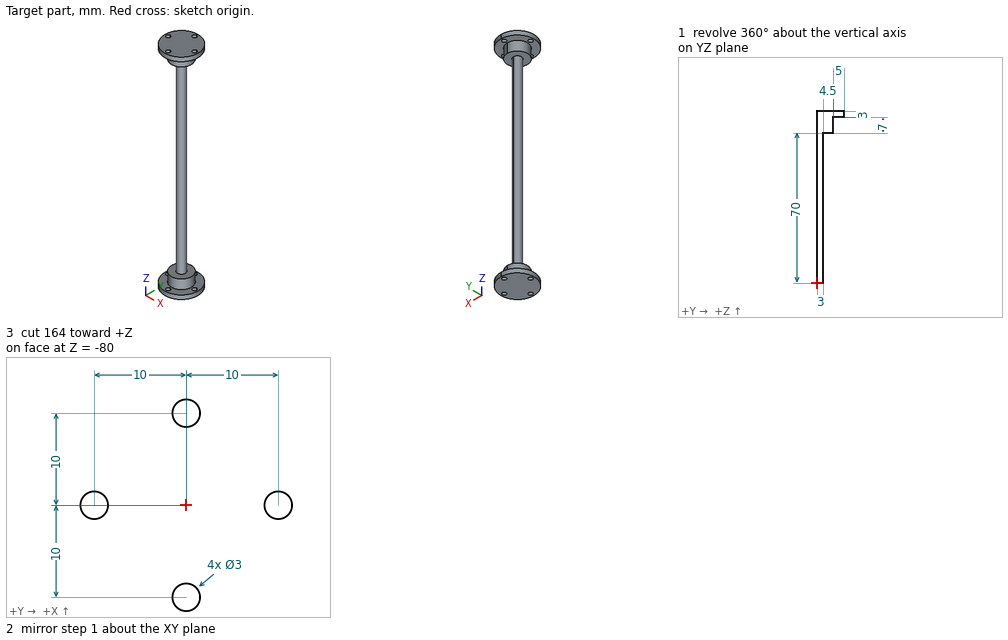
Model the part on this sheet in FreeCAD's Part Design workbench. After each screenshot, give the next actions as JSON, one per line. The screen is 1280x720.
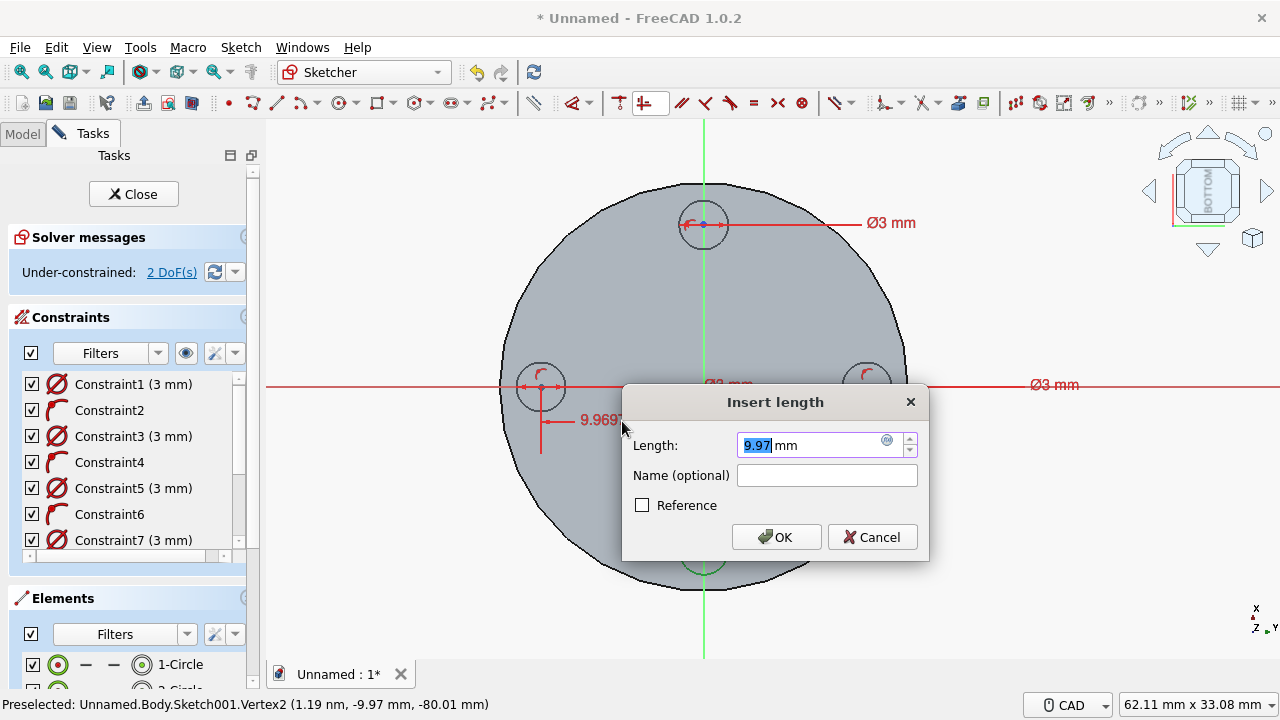
{"action": "type", "text": "10"}
{"action": "key", "text": "Return"}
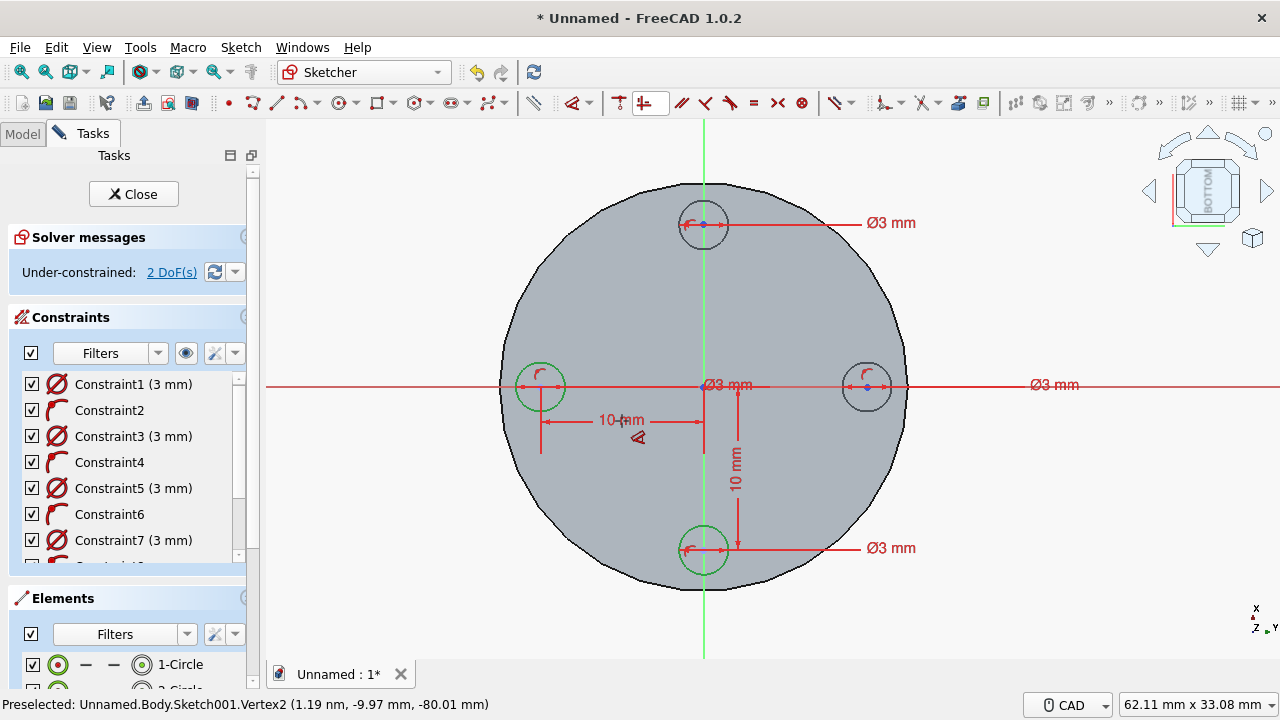
{"action": "left_click", "coordinate": [704, 225]}
{"action": "left_click", "coordinate": [738, 306]}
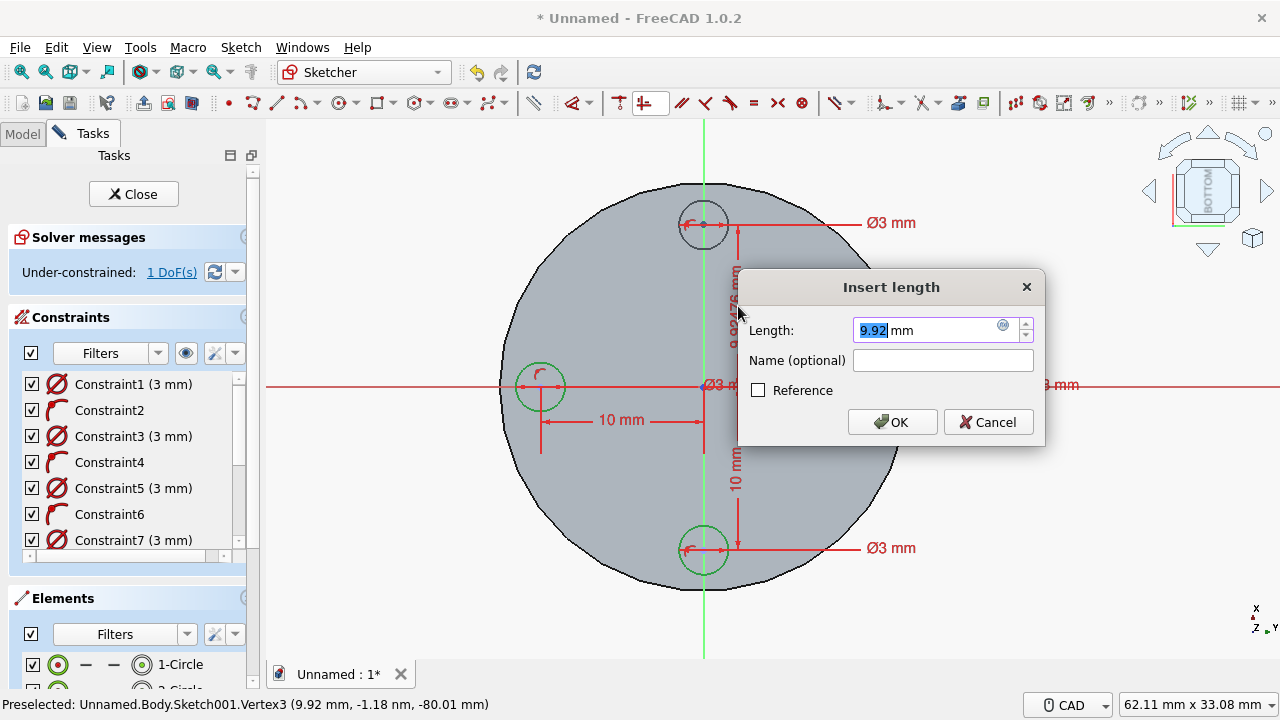
{"action": "type", "text": "10"}
{"action": "key", "text": "Return"}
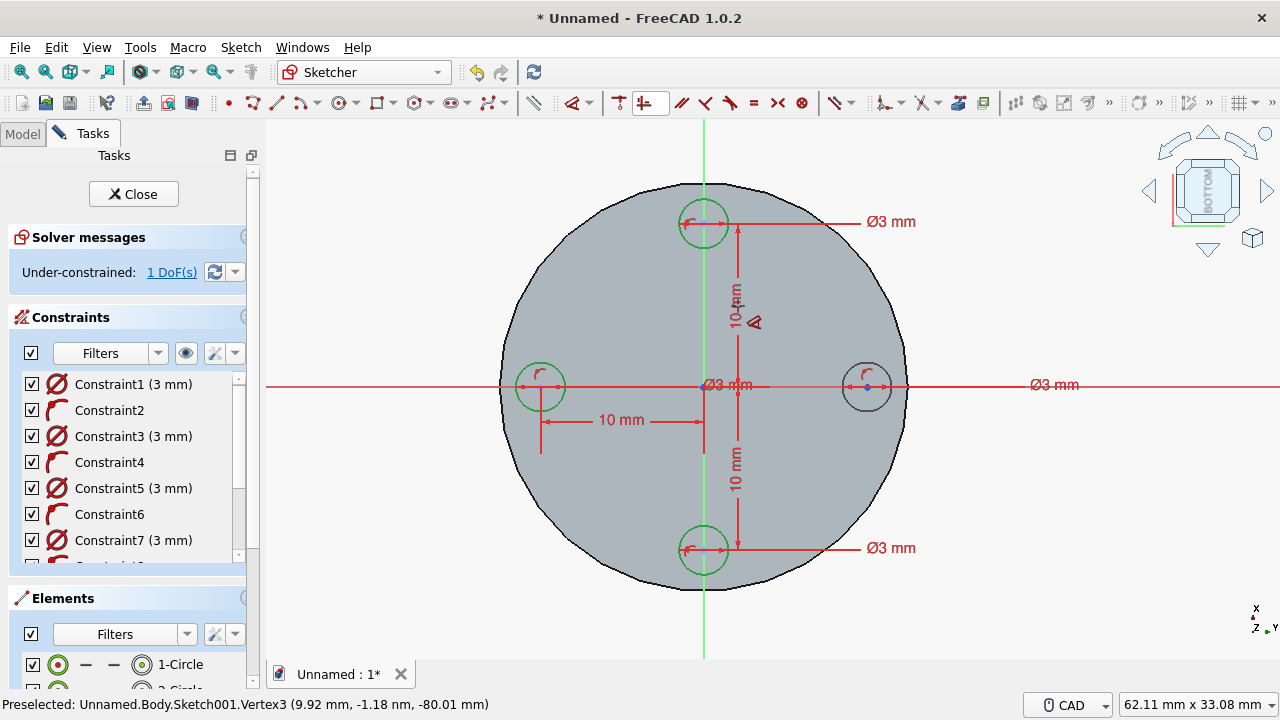
{"action": "left_click", "coordinate": [867, 387]}
{"action": "left_click", "coordinate": [785, 353]}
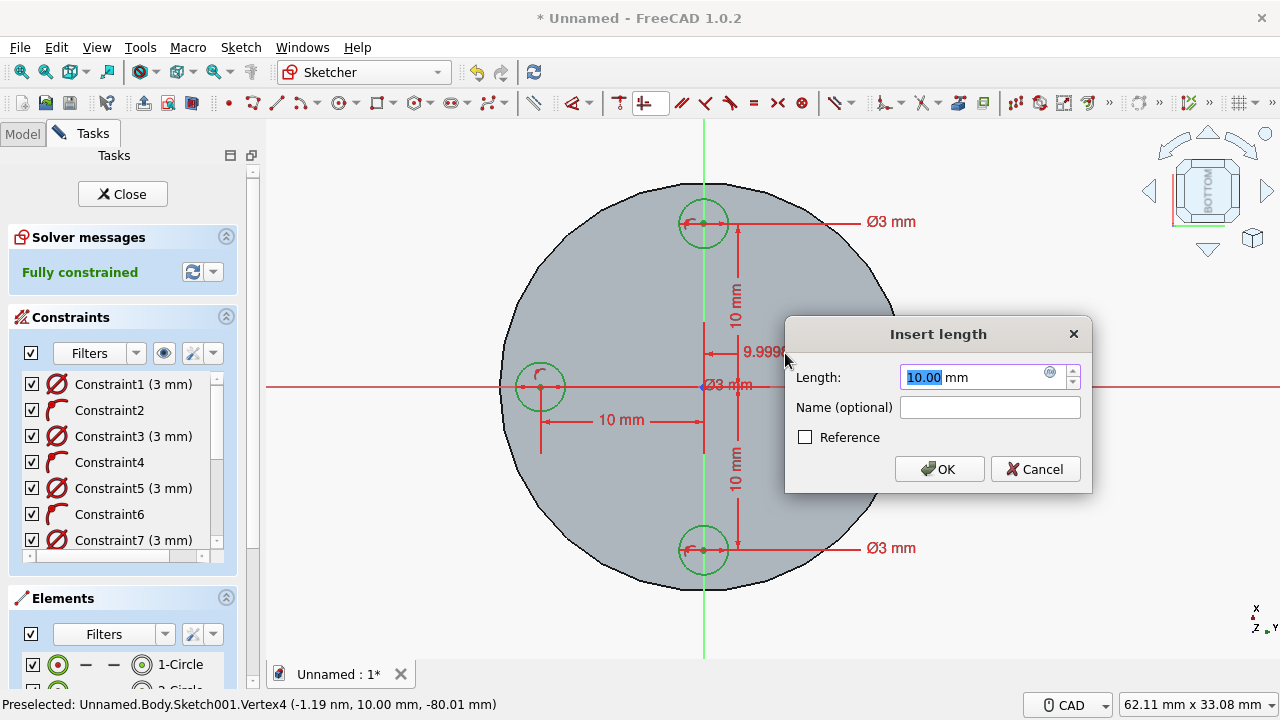
{"action": "type", "text": "10"}
{"action": "key", "text": "Return"}
{"action": "key", "text": "Escape"}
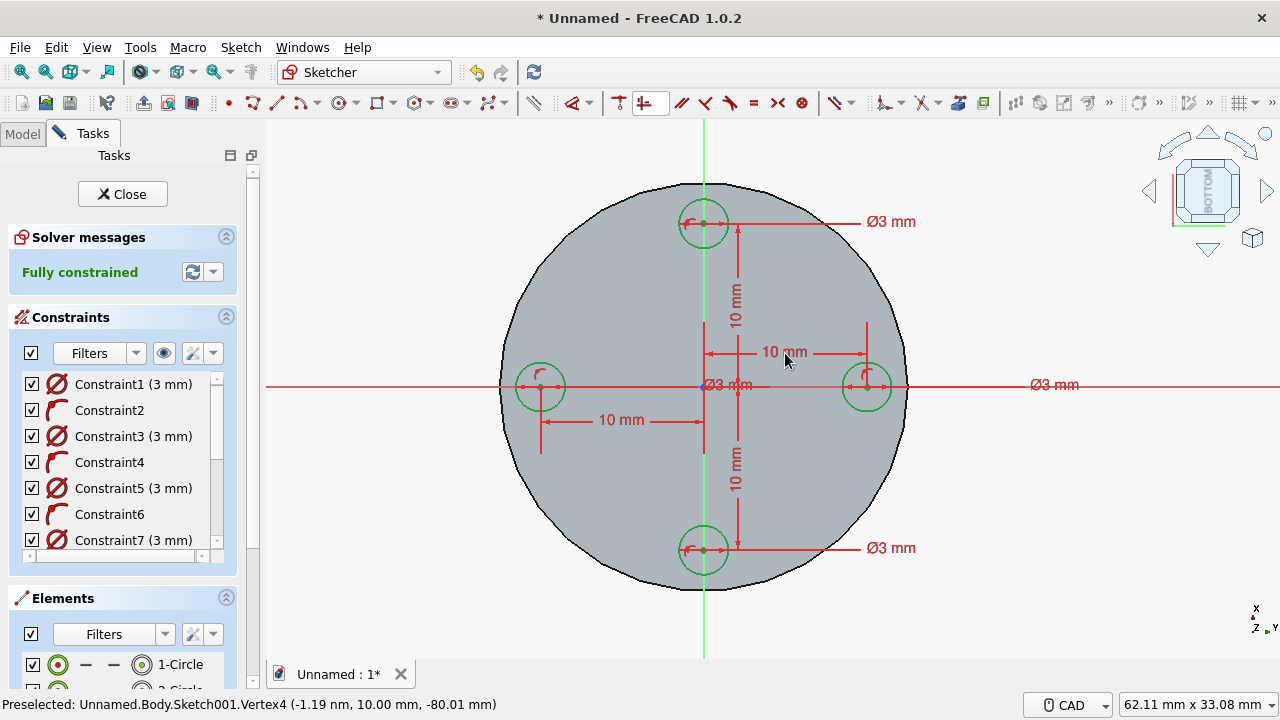
{"action": "left_click", "coordinate": [123, 194]}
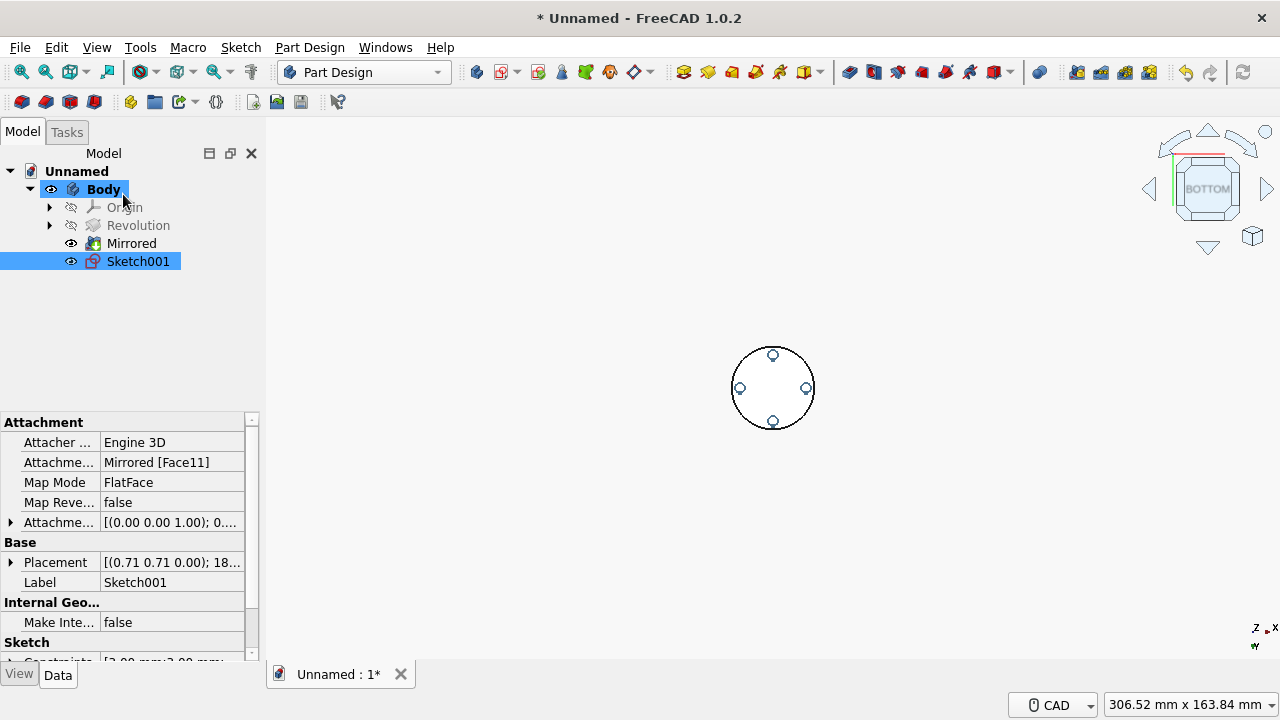
{"action": "left_click", "coordinate": [850, 72]}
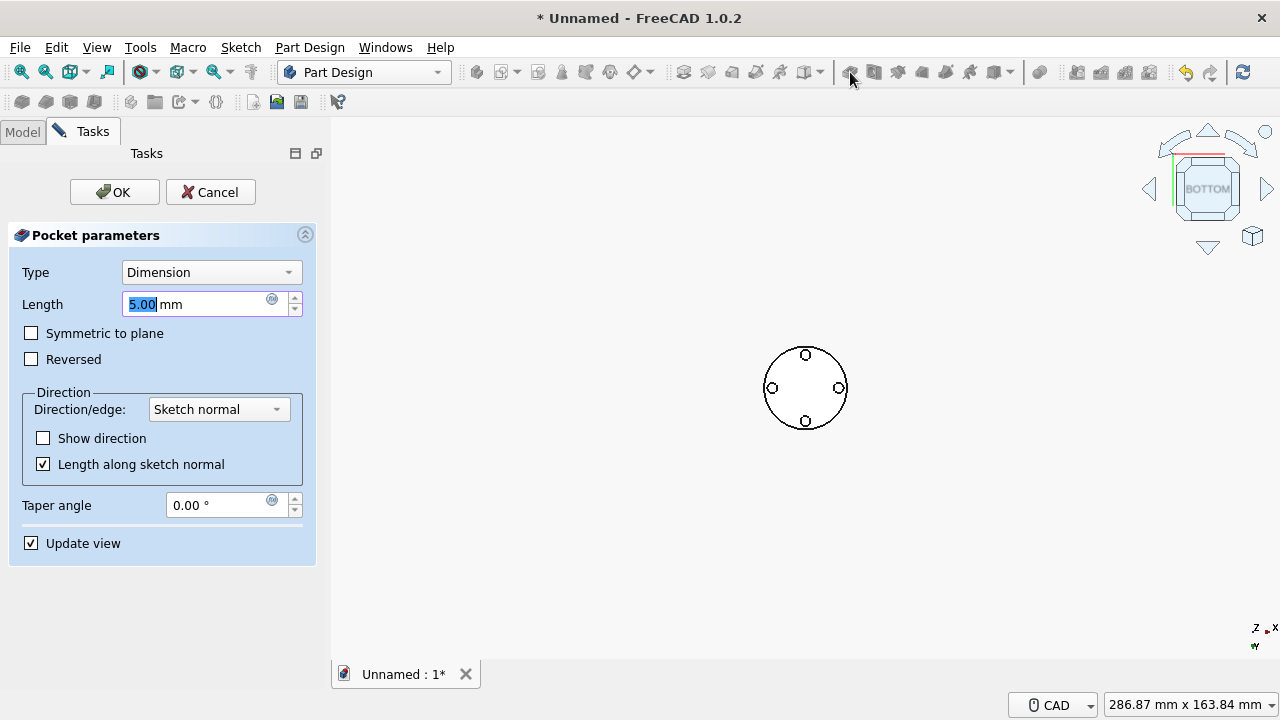
{"action": "type", "text": "164"}
{"action": "key", "text": "Tab"}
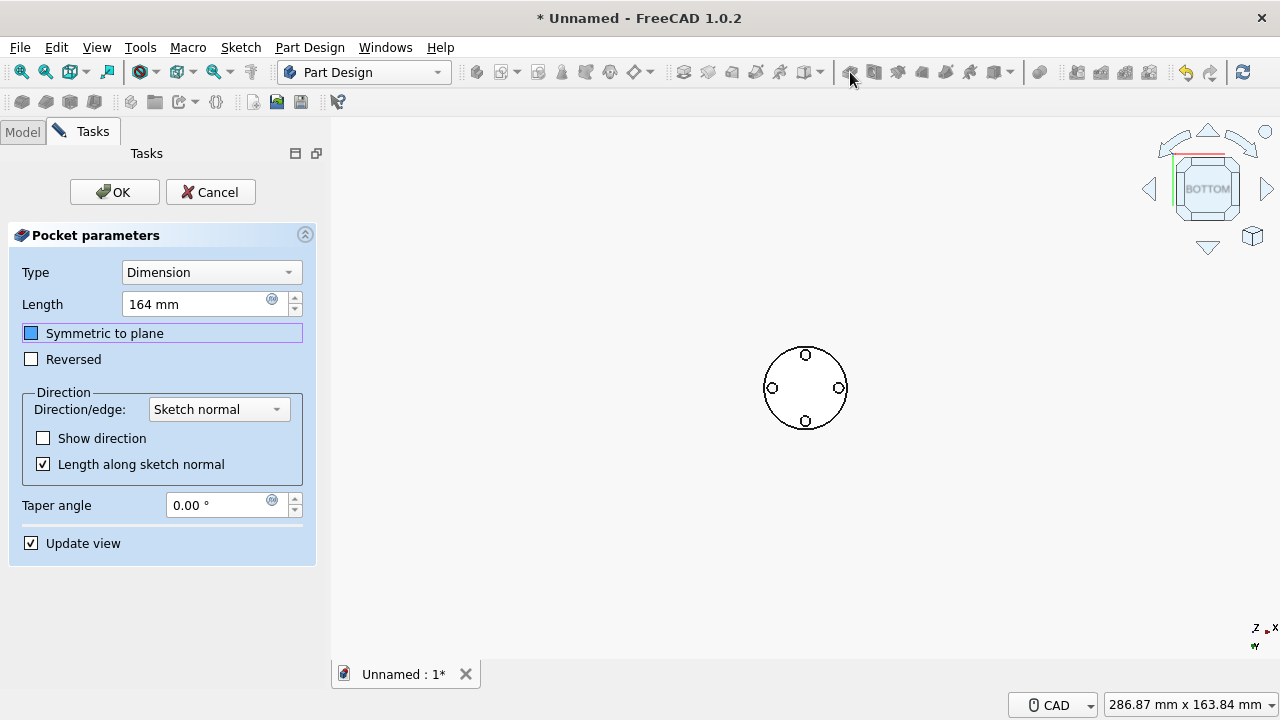
{"action": "left_click", "coordinate": [115, 192]}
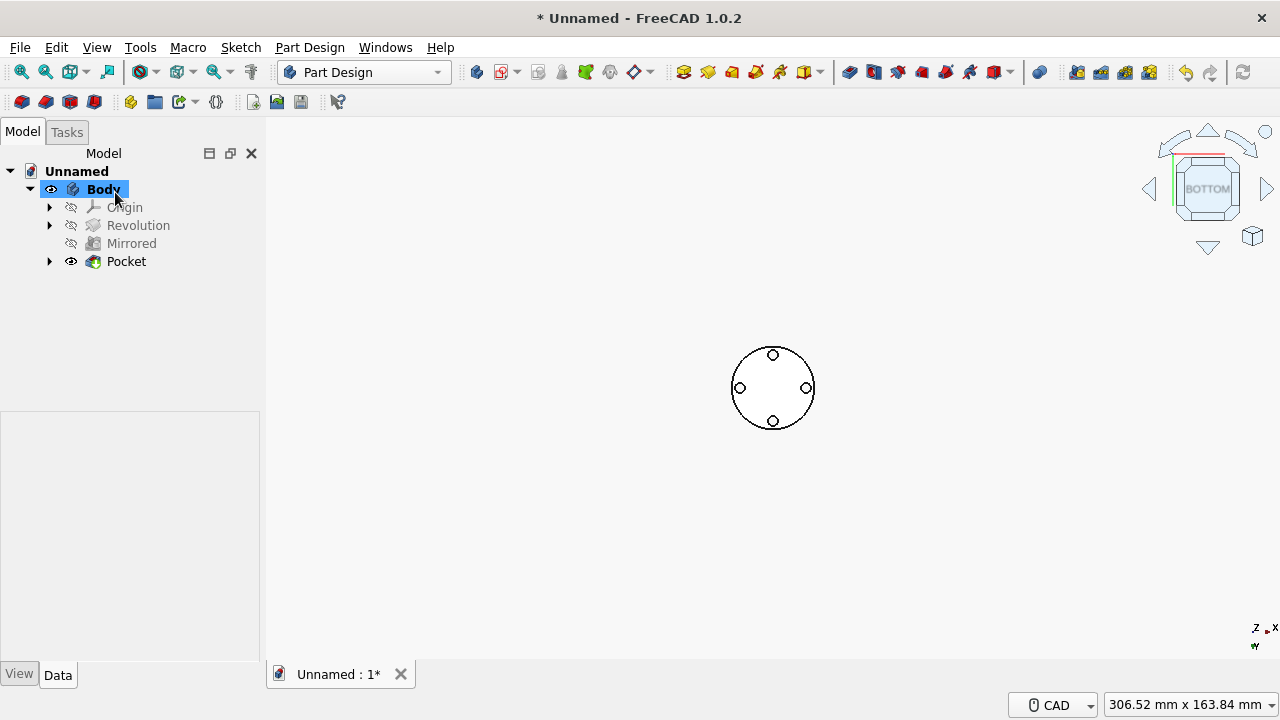
{"action": "key", "text": "0"}